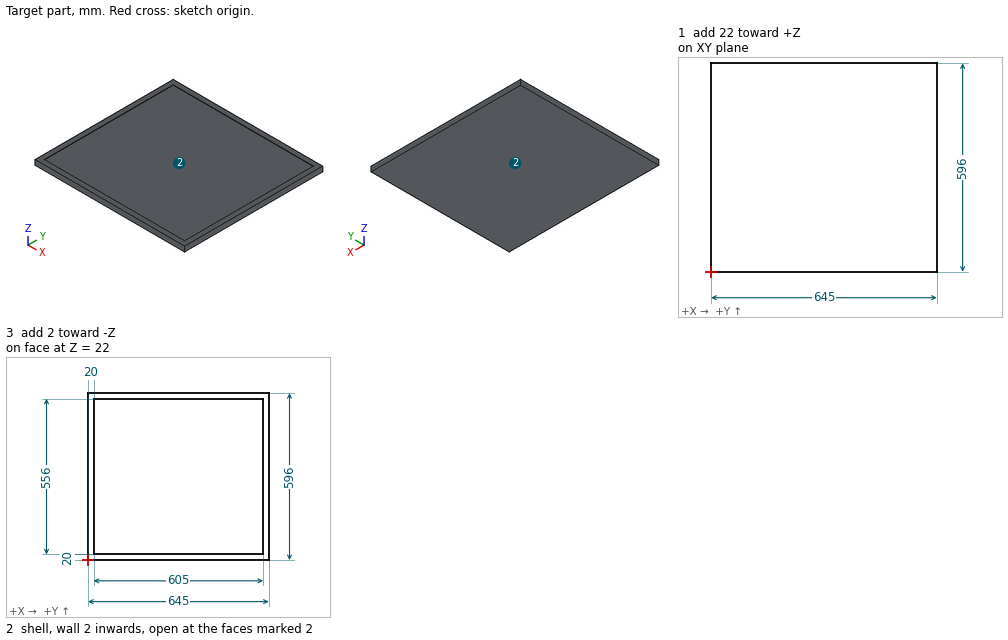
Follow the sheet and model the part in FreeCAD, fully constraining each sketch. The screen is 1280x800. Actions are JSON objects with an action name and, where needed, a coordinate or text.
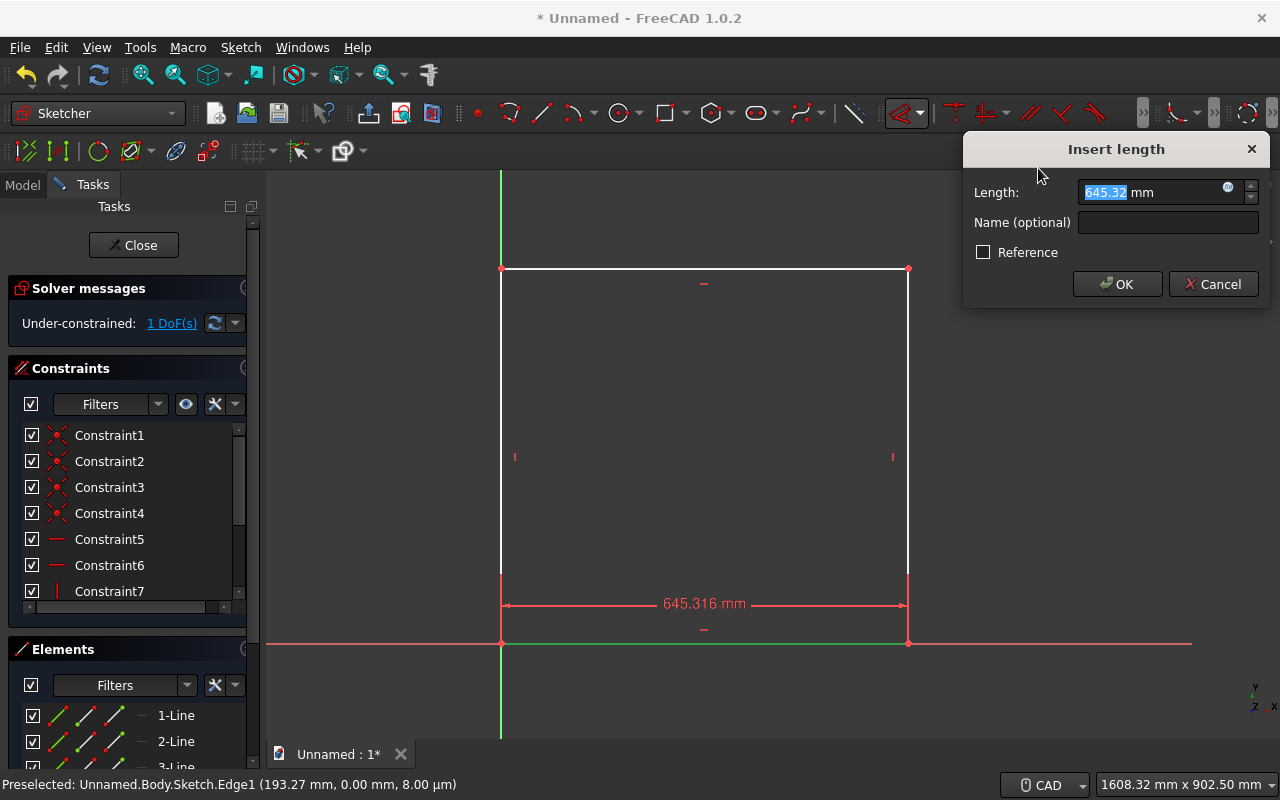
{"action": "type", "text": "645"}
{"action": "key", "text": "Return"}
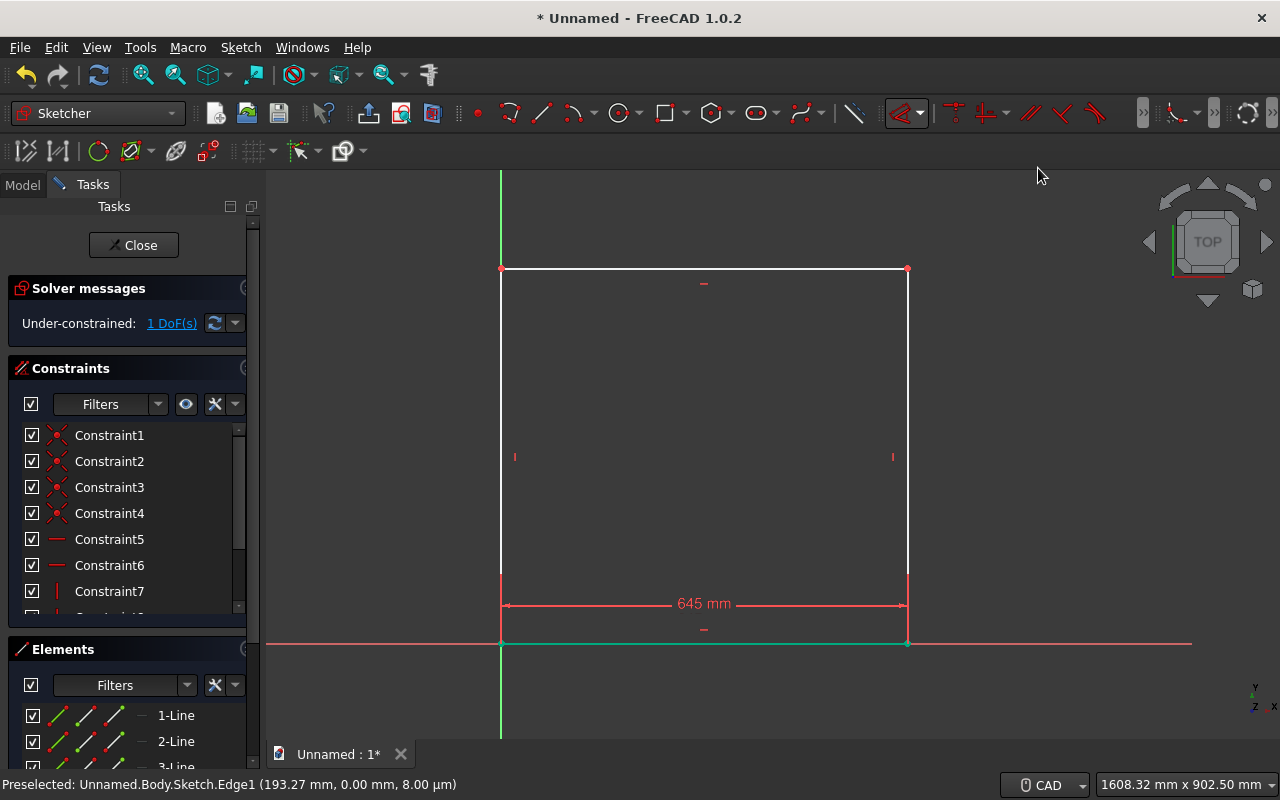
{"action": "left_click", "coordinate": [908, 531]}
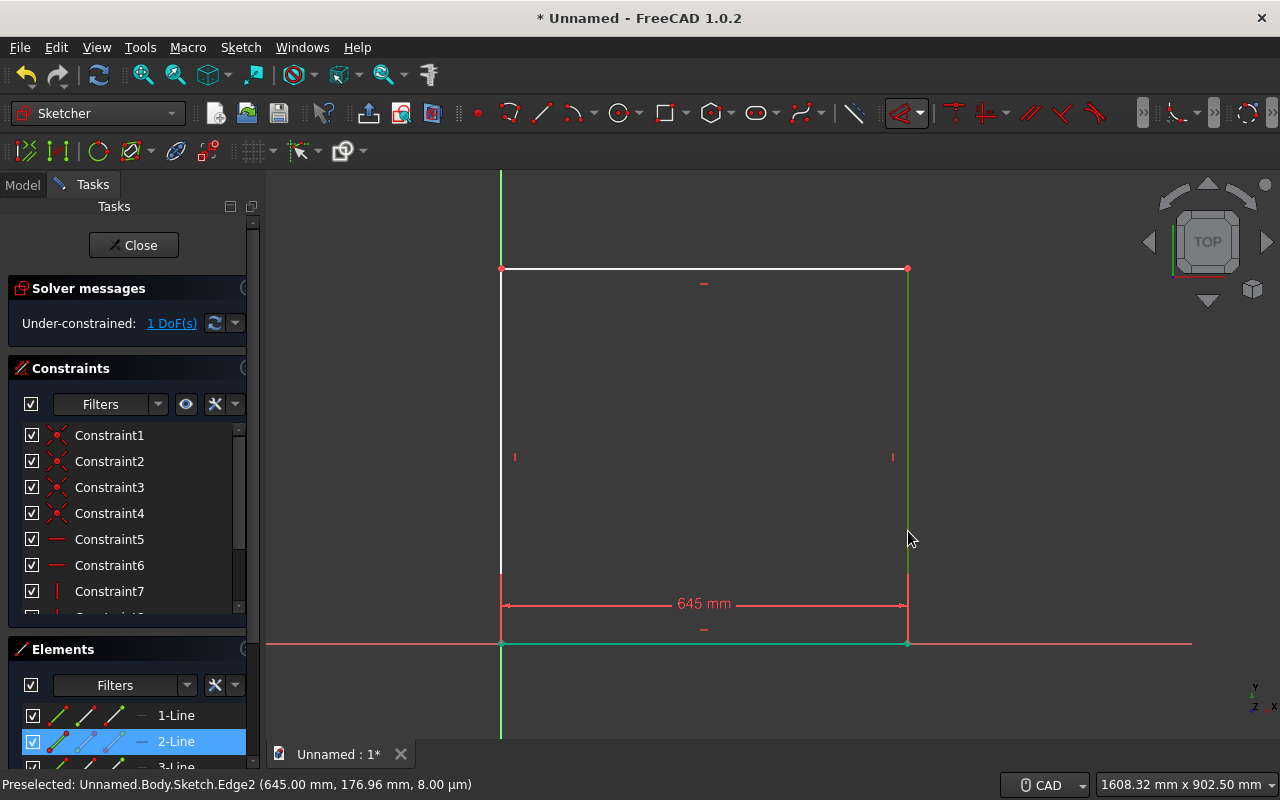
{"action": "key", "text": "i"}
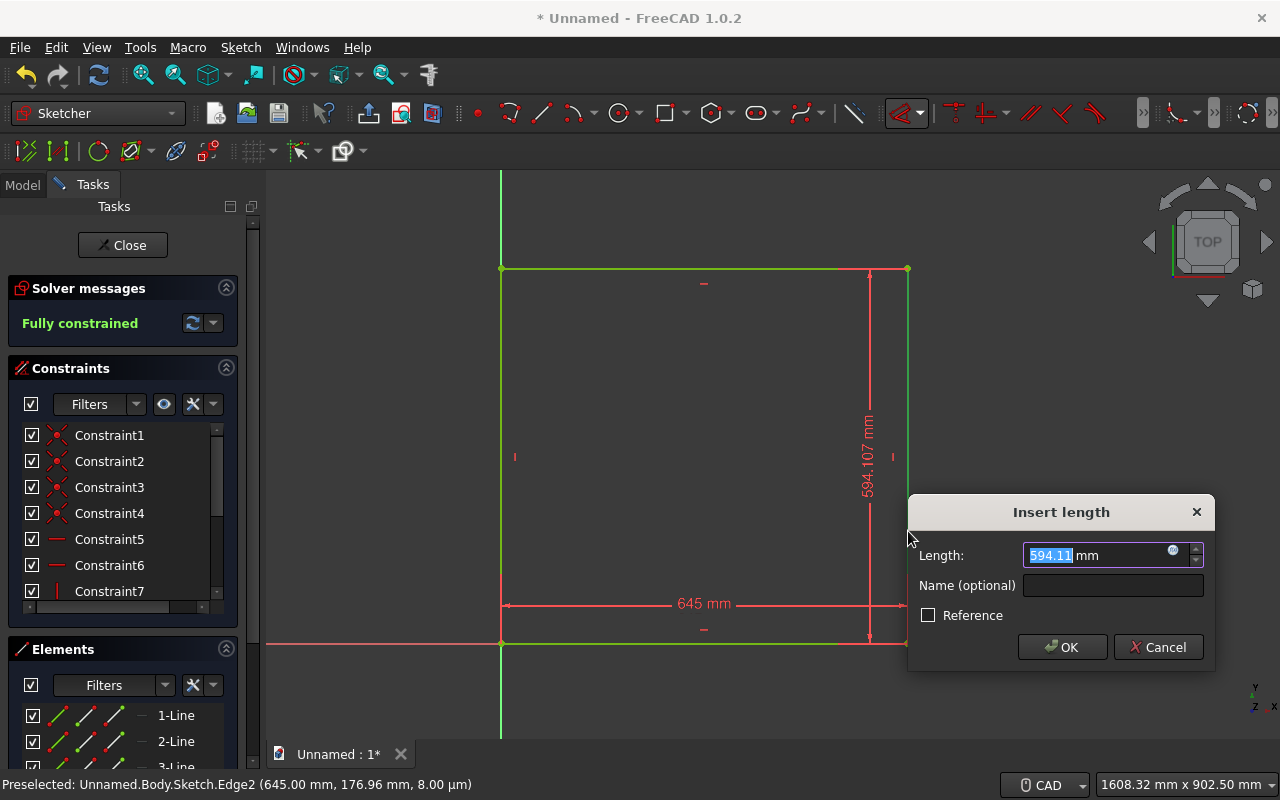
{"action": "type", "text": "596"}
{"action": "key", "text": "Return"}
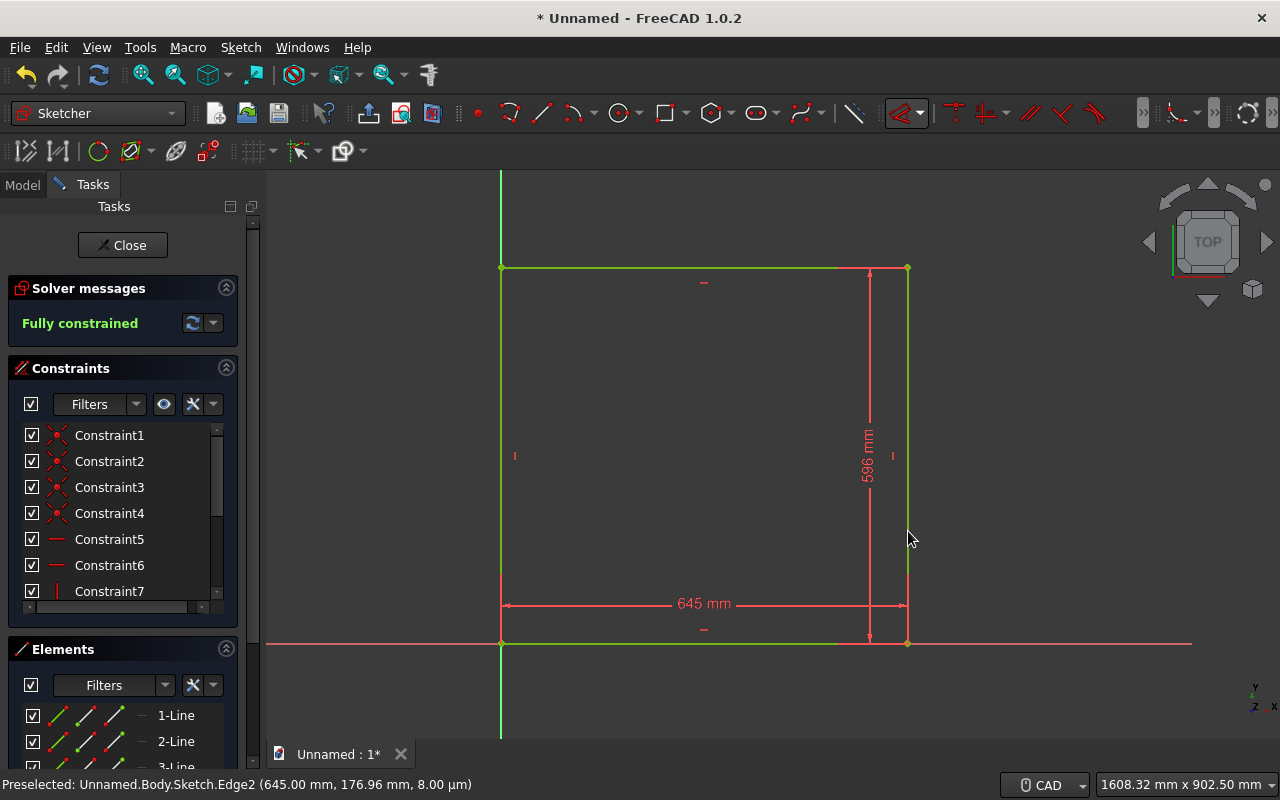
{"action": "left_click", "coordinate": [123, 245]}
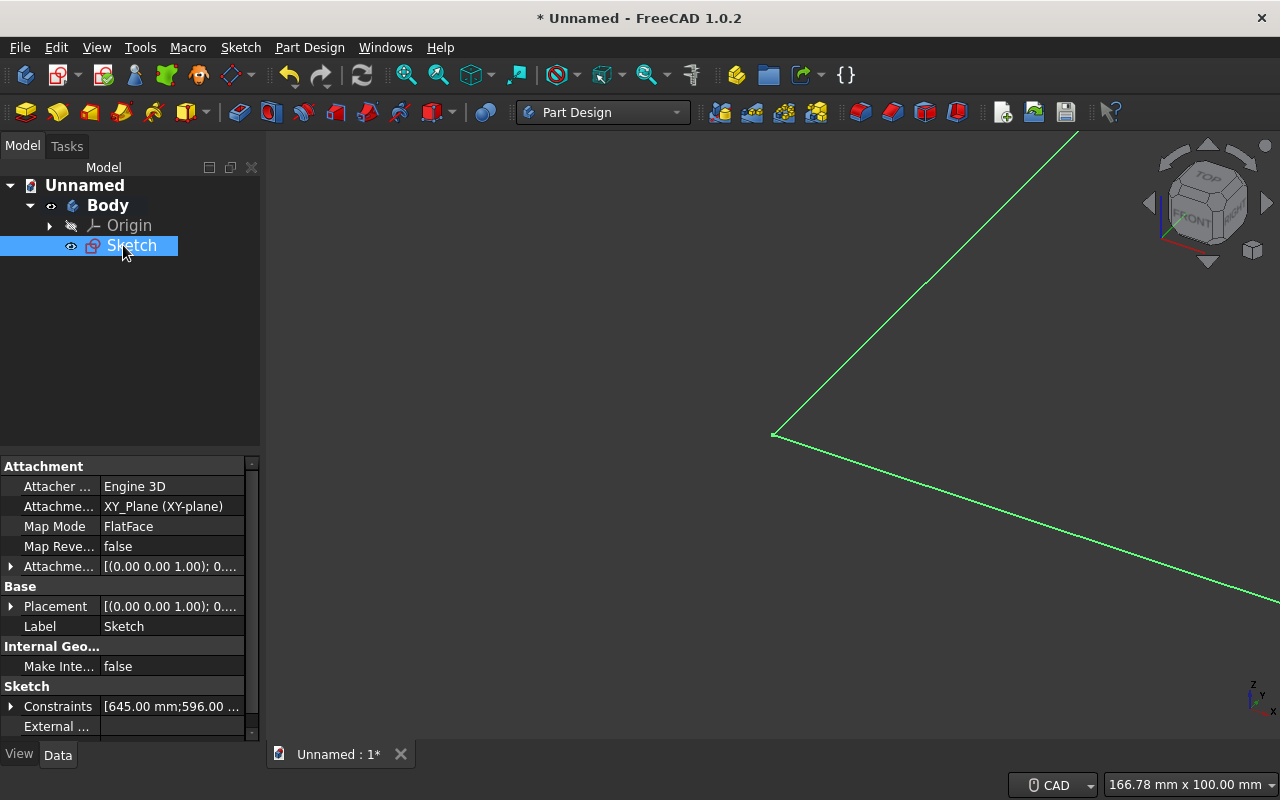
{"action": "left_click", "coordinate": [26, 112]}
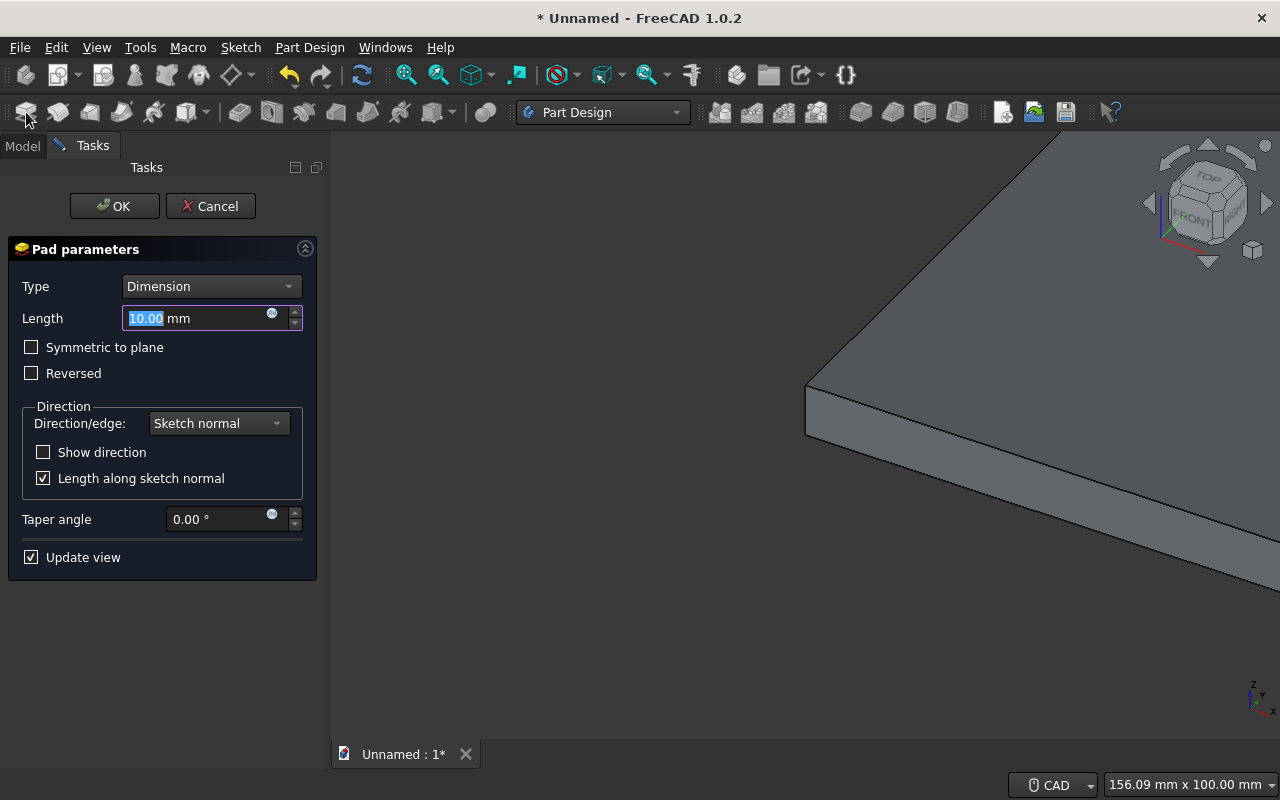
{"action": "type", "text": "22"}
{"action": "key", "text": "Tab"}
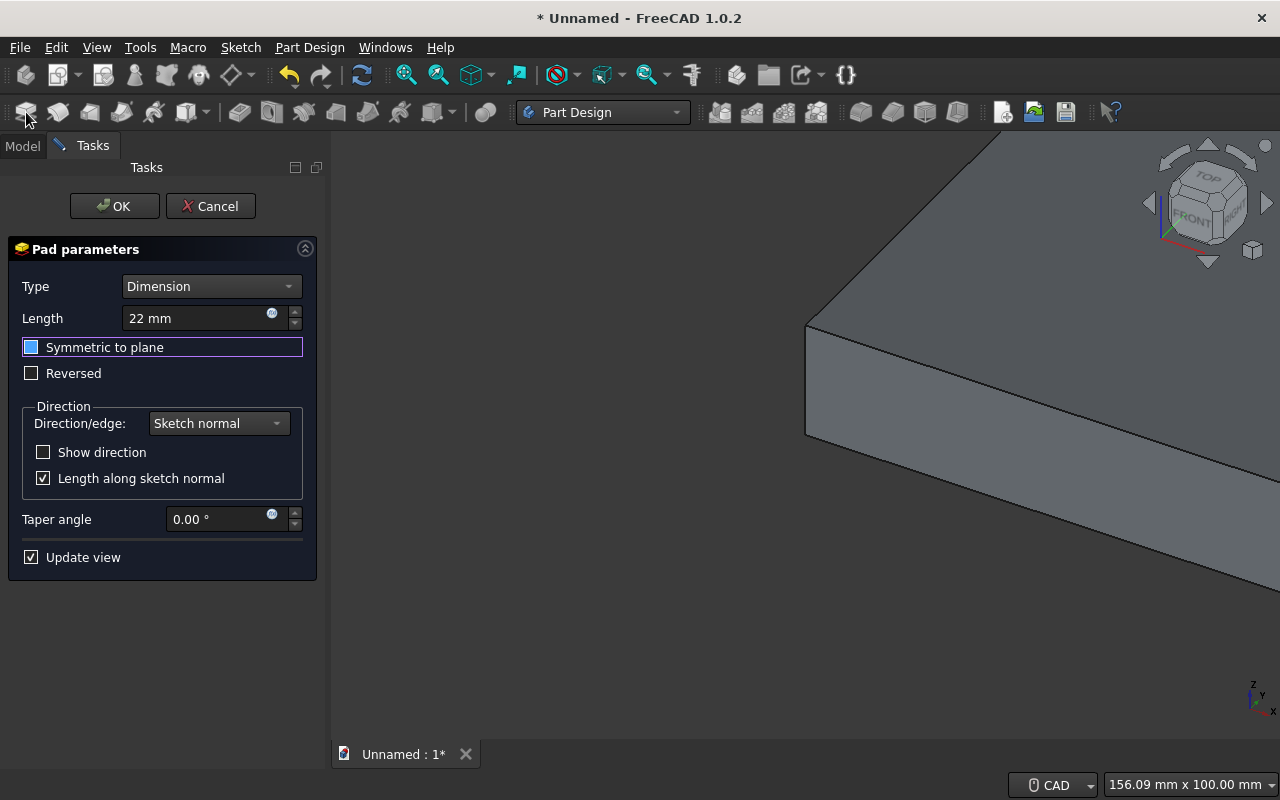
{"action": "left_click", "coordinate": [115, 206]}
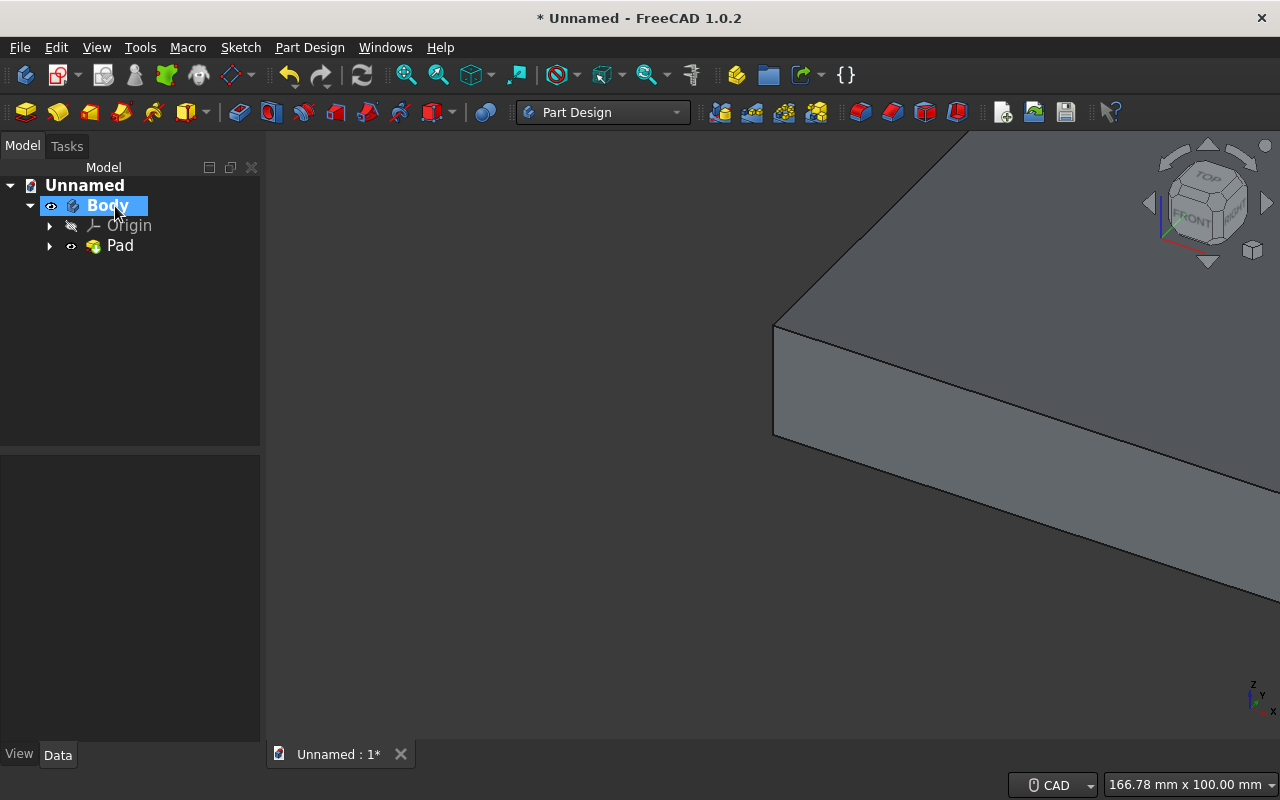
{"action": "key", "text": "v f"}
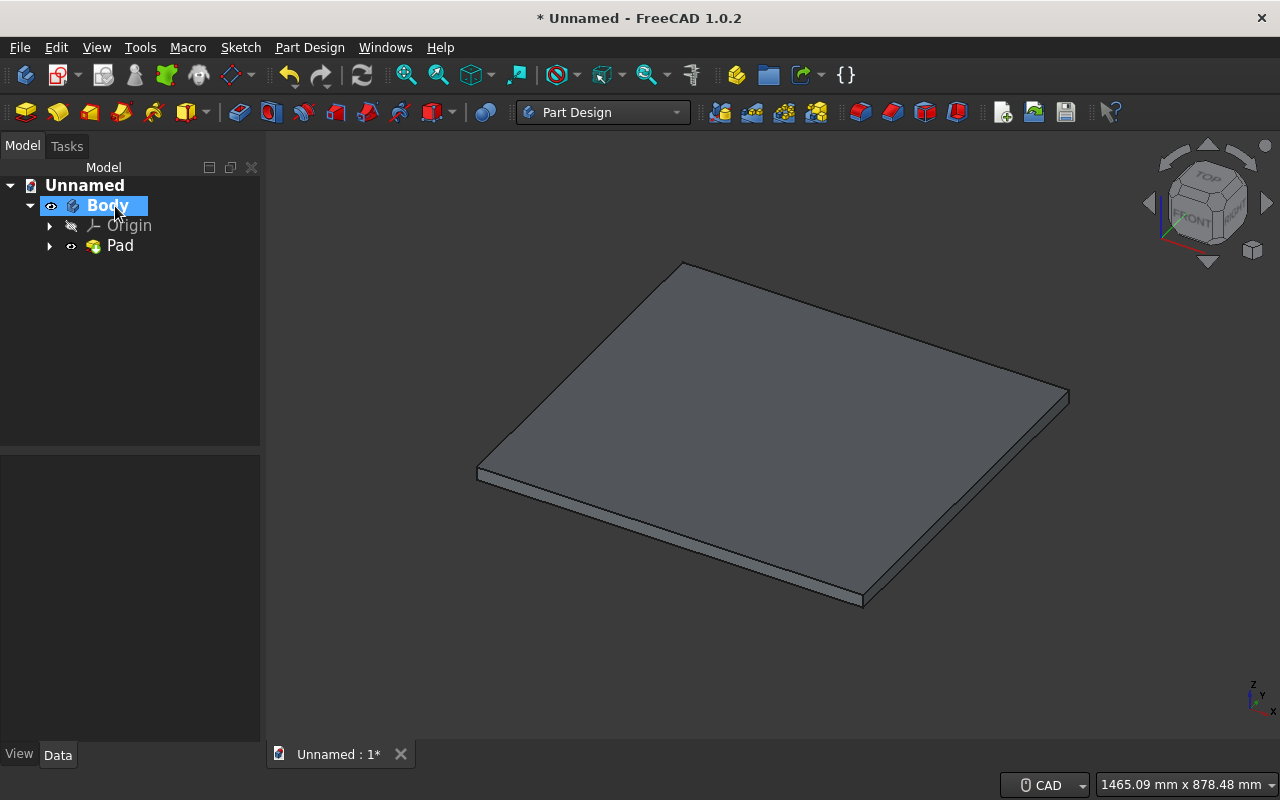
{"action": "left_click", "coordinate": [773, 428]}